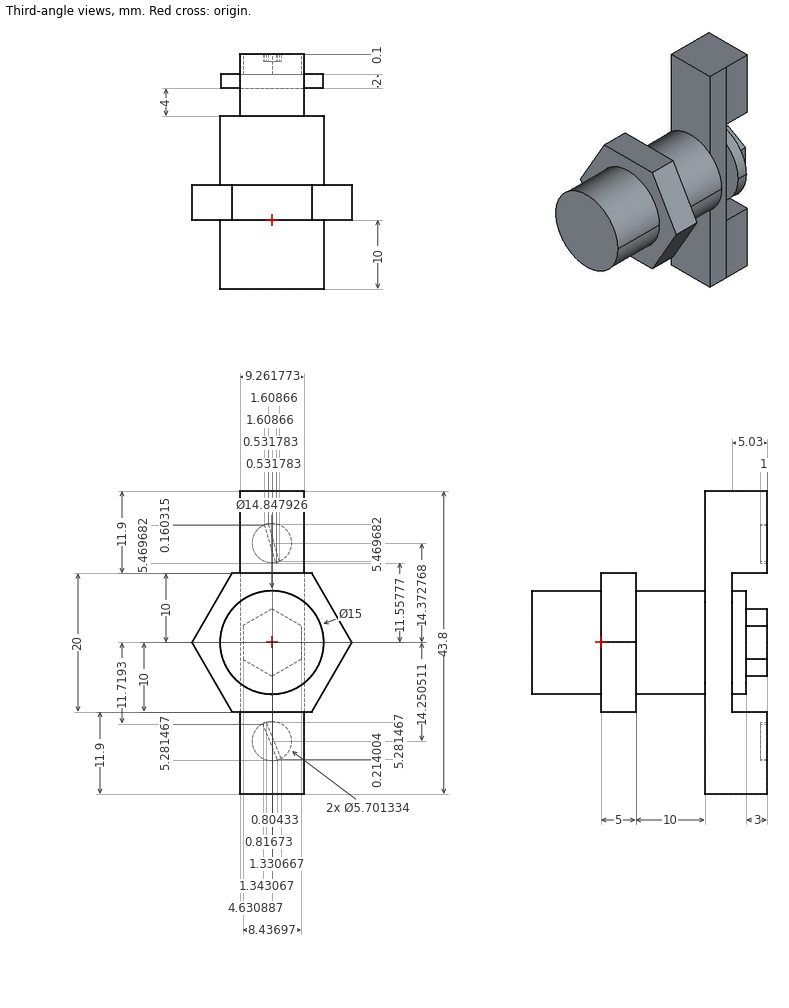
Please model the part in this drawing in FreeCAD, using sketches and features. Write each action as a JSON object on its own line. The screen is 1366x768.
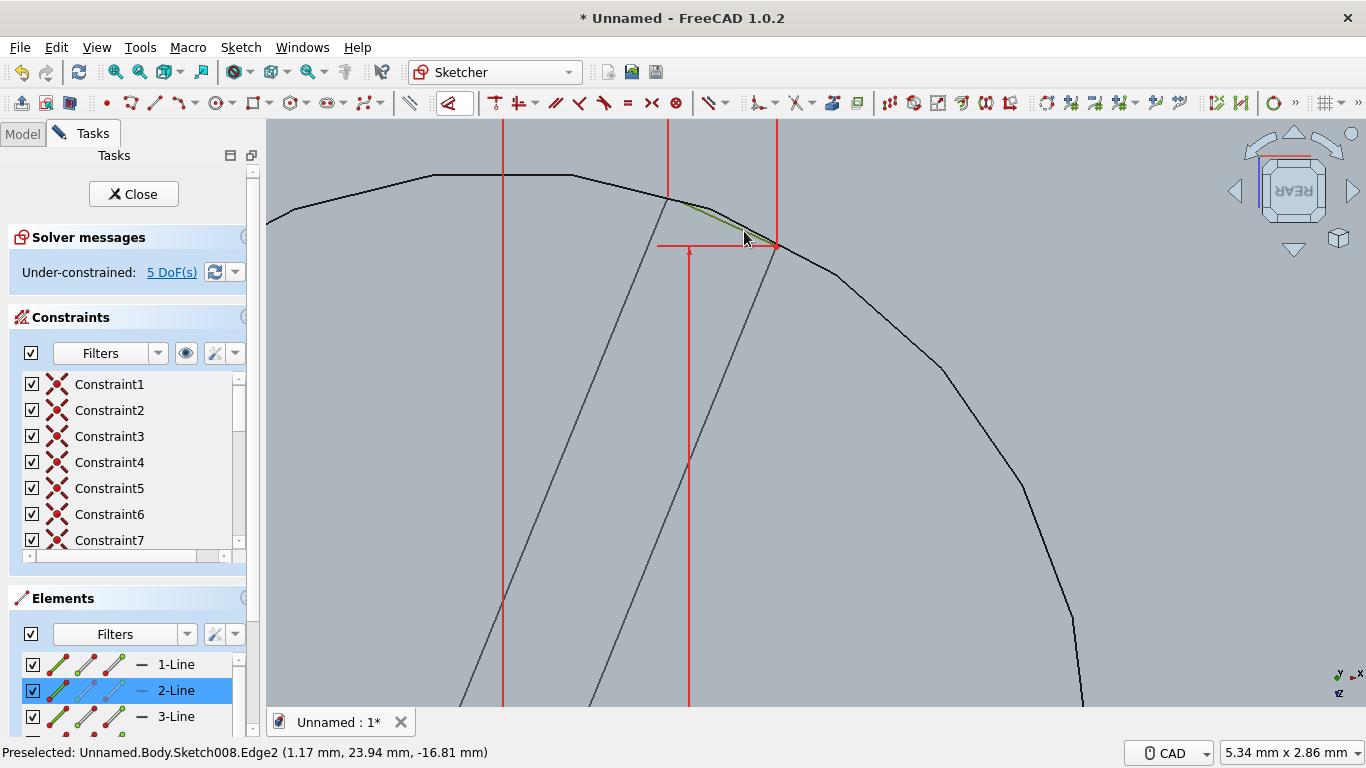
{"action": "left_click", "coordinate": [468, 104]}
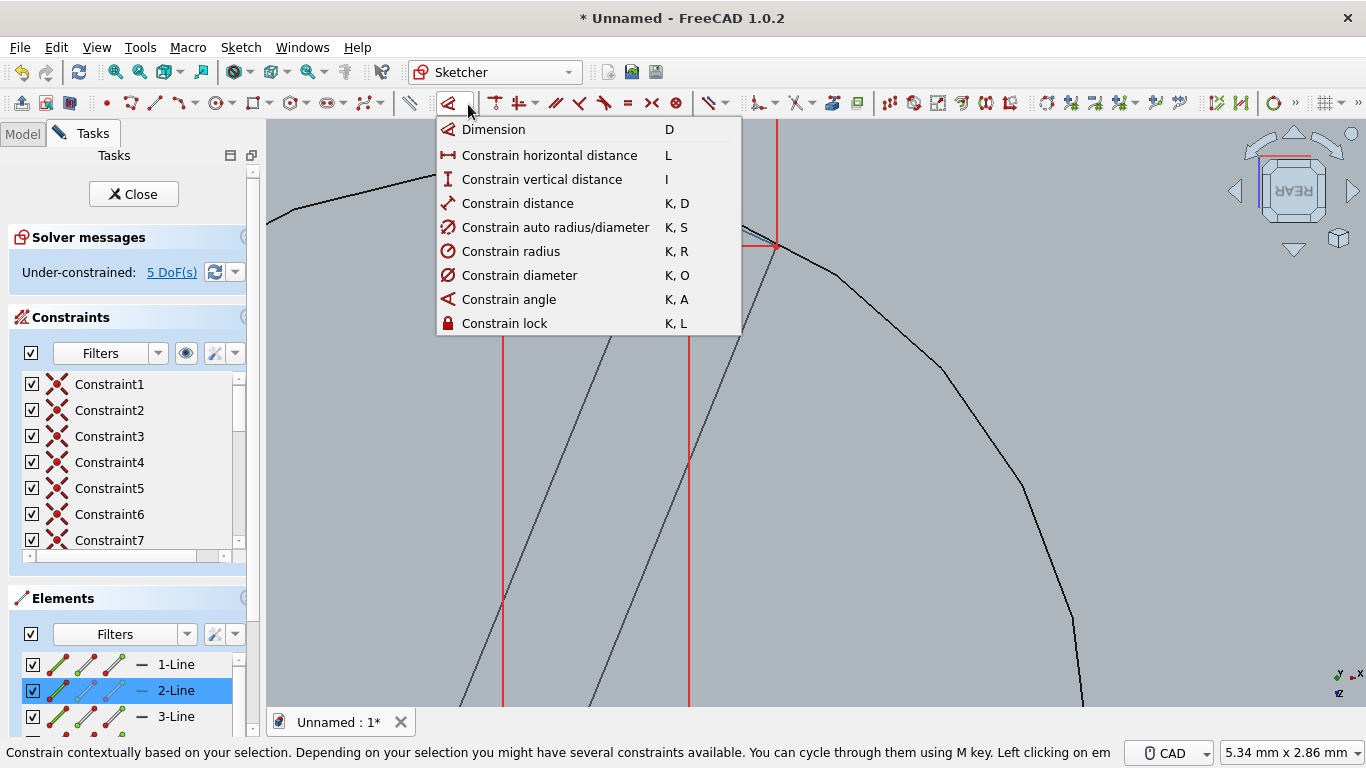
{"action": "left_click", "coordinate": [589, 179]}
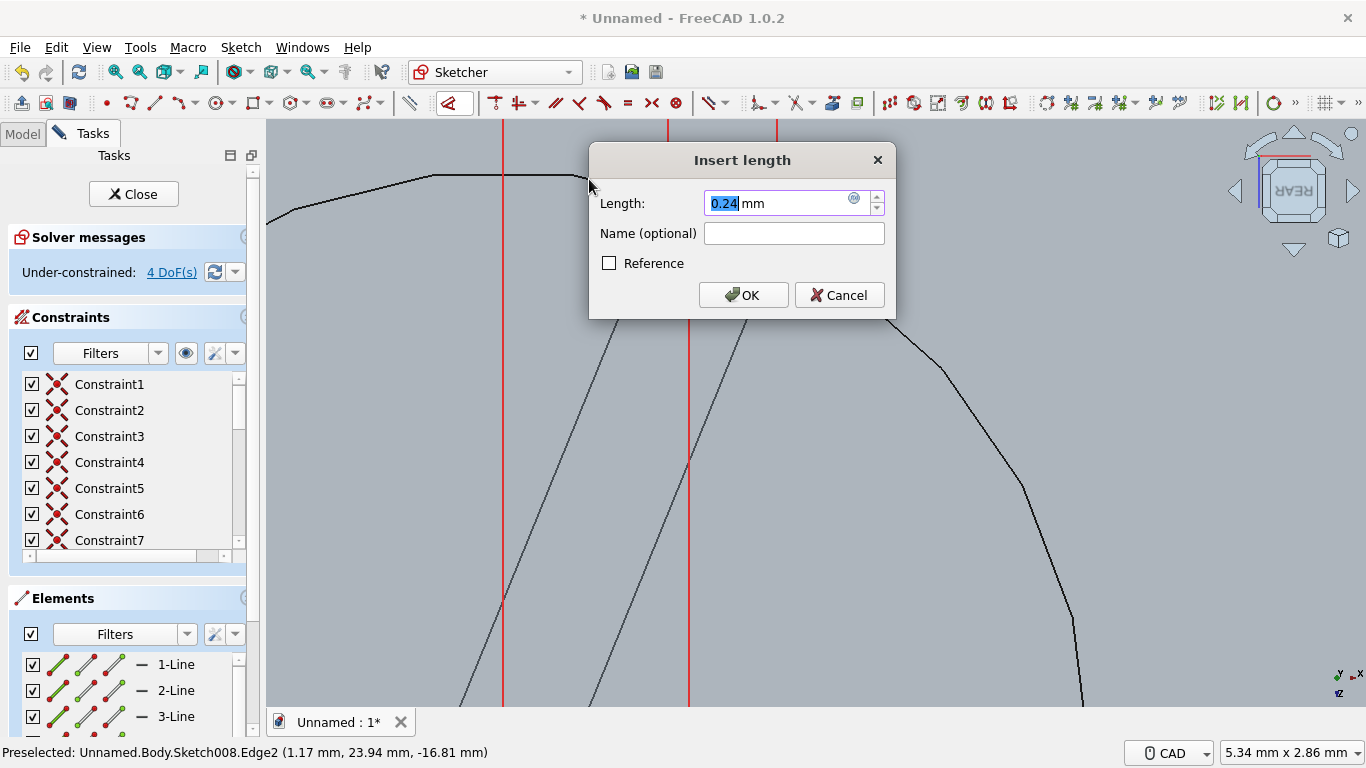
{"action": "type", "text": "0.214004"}
{"action": "key", "text": "Return"}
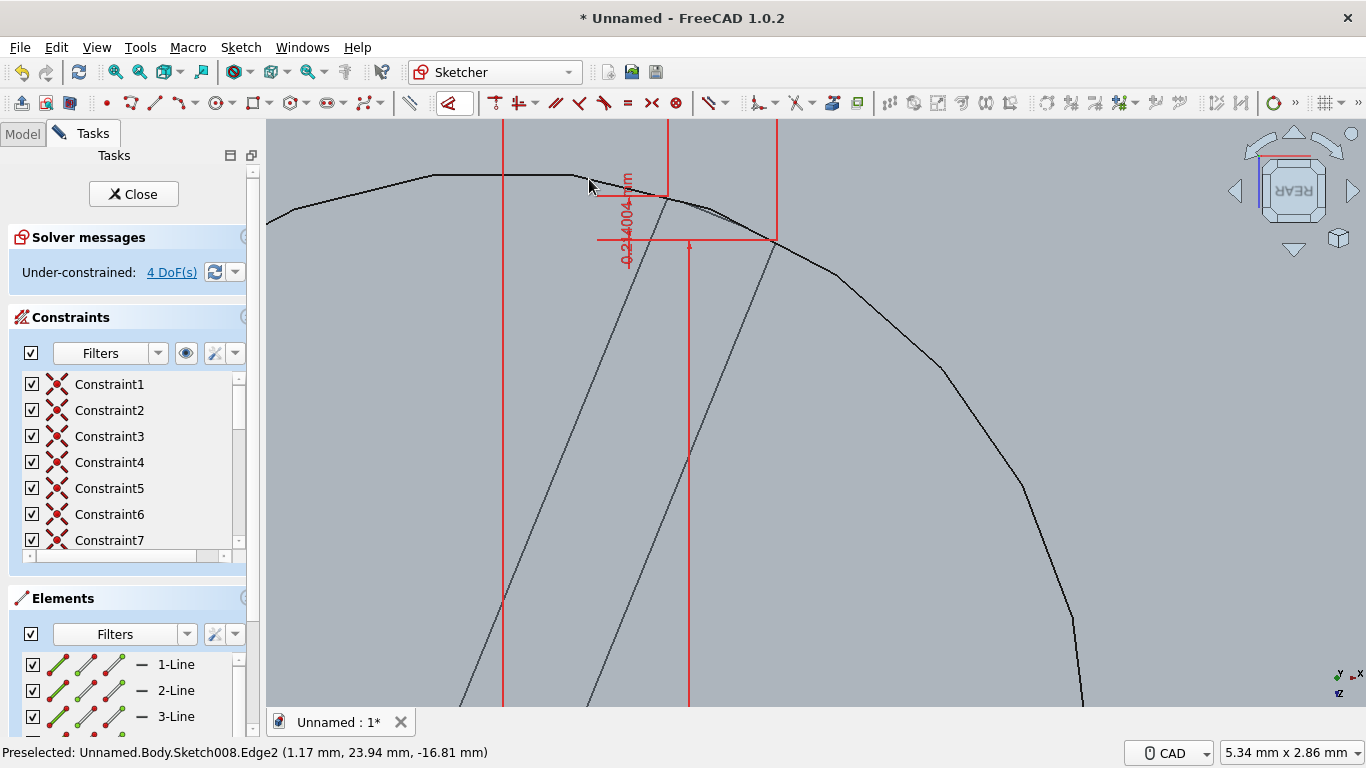
{"action": "left_click", "coordinate": [536, 521]}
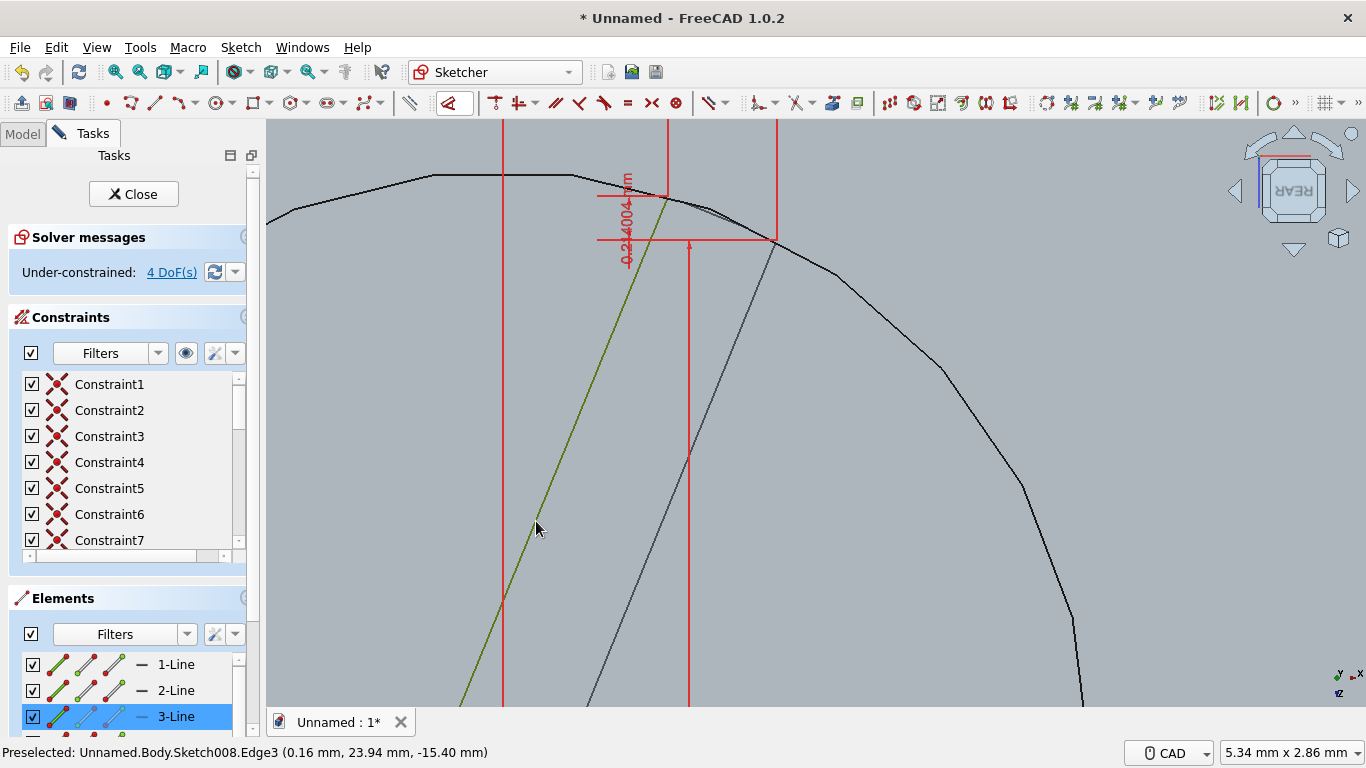
{"action": "key", "text": "i"}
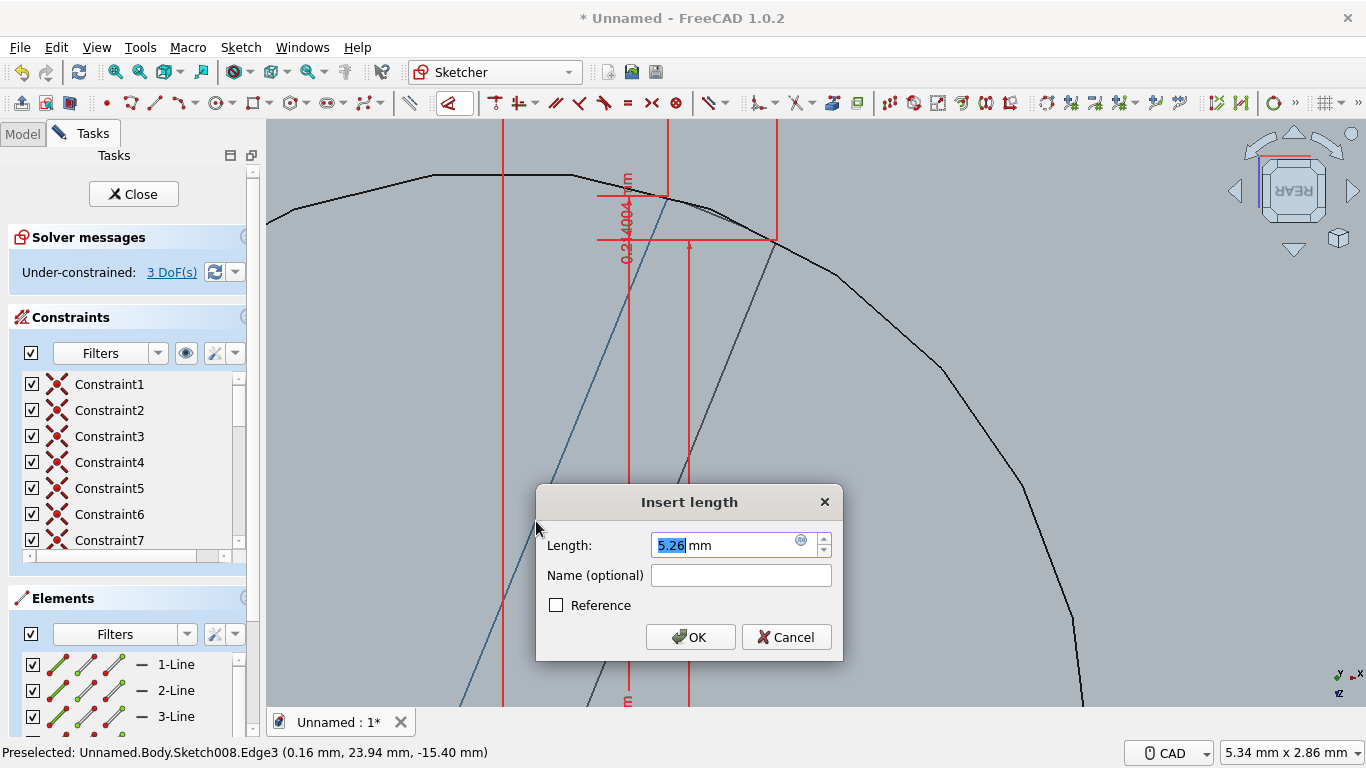
{"action": "type", "text": "5.281467"}
{"action": "key", "text": "Return"}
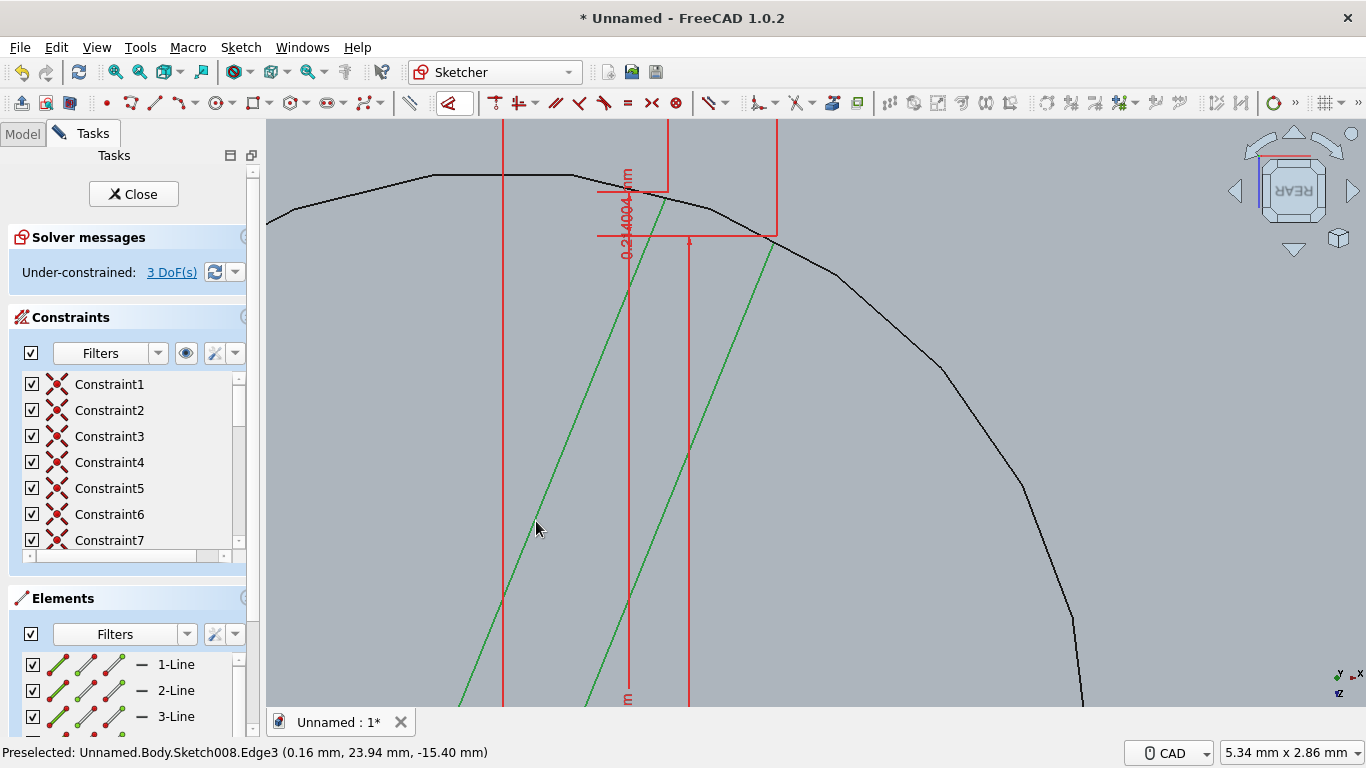
{"action": "scroll", "coordinate": [760, 240], "scroll_direction": "down", "scroll_amount": 15}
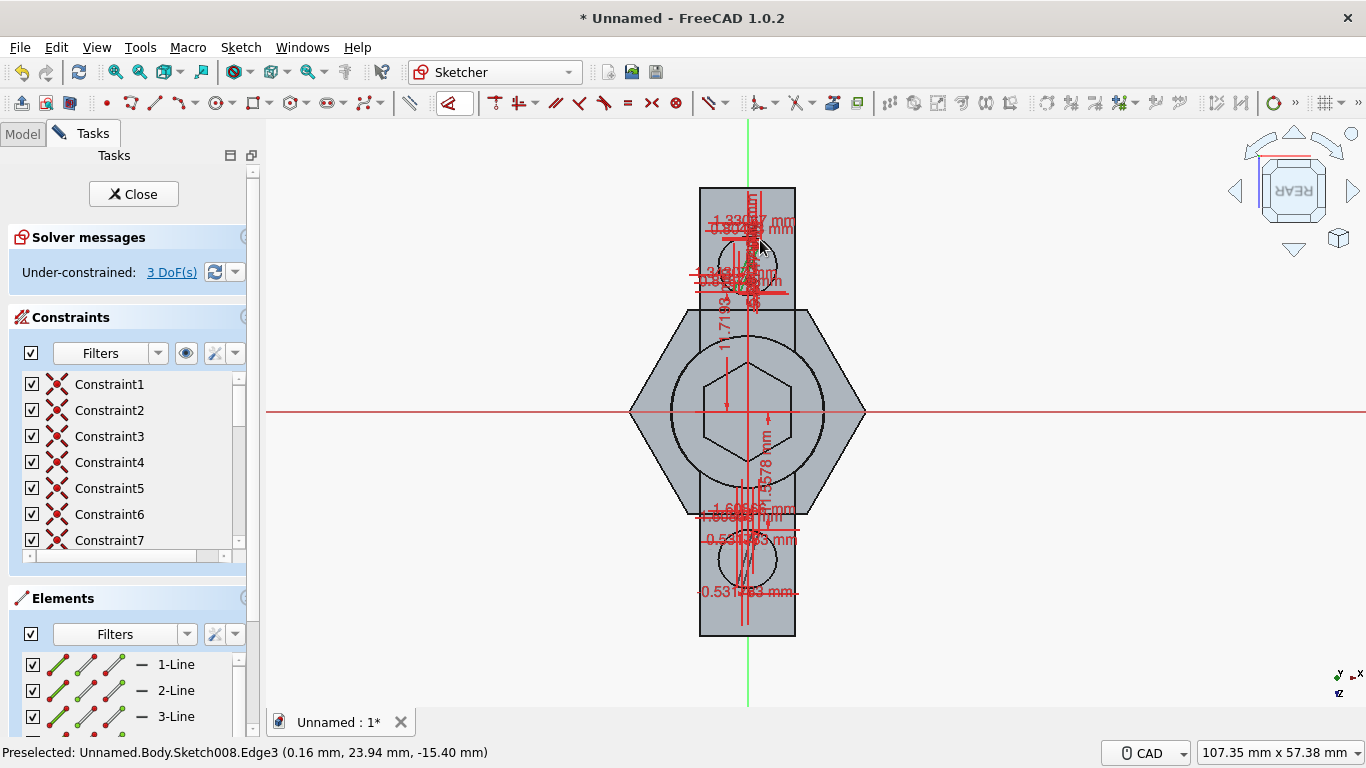
{"action": "scroll", "coordinate": [748, 547], "scroll_direction": "up", "scroll_amount": 14}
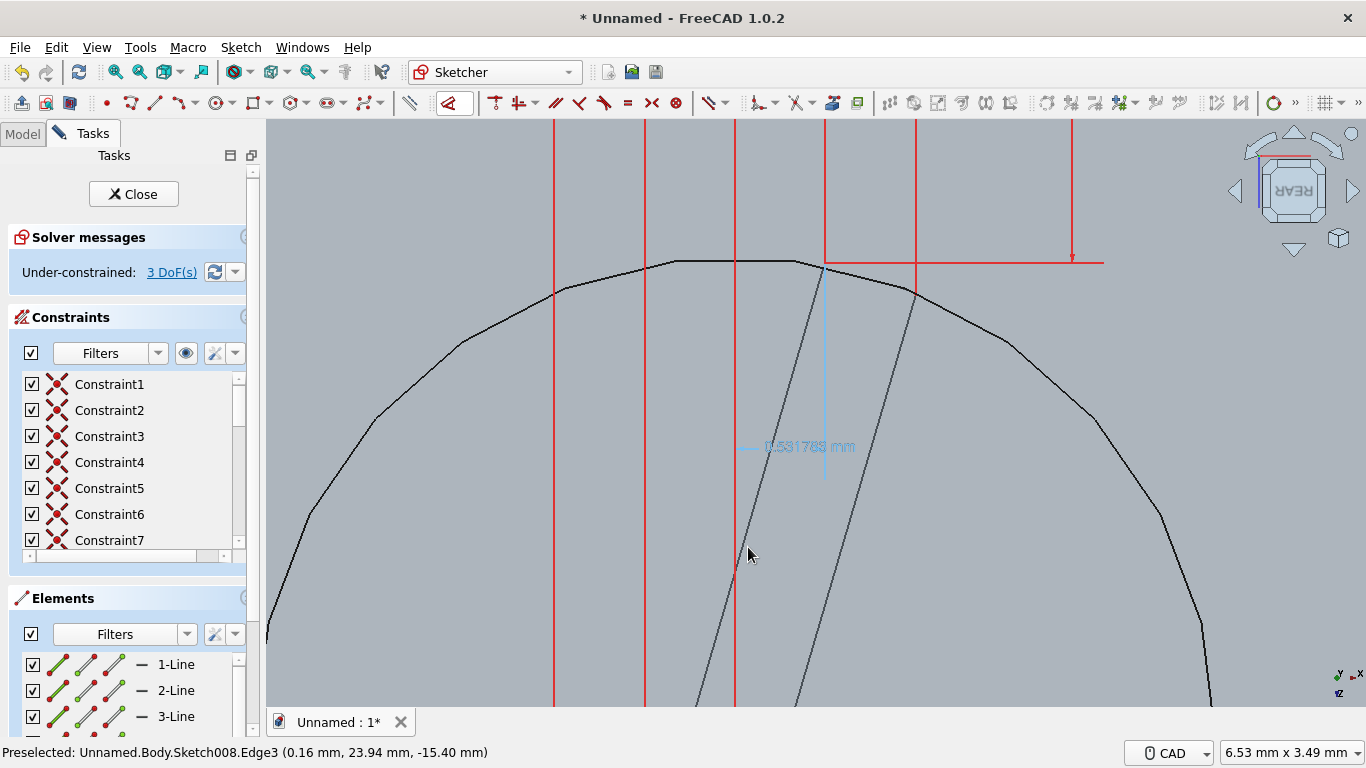
{"action": "left_click", "coordinate": [743, 544]}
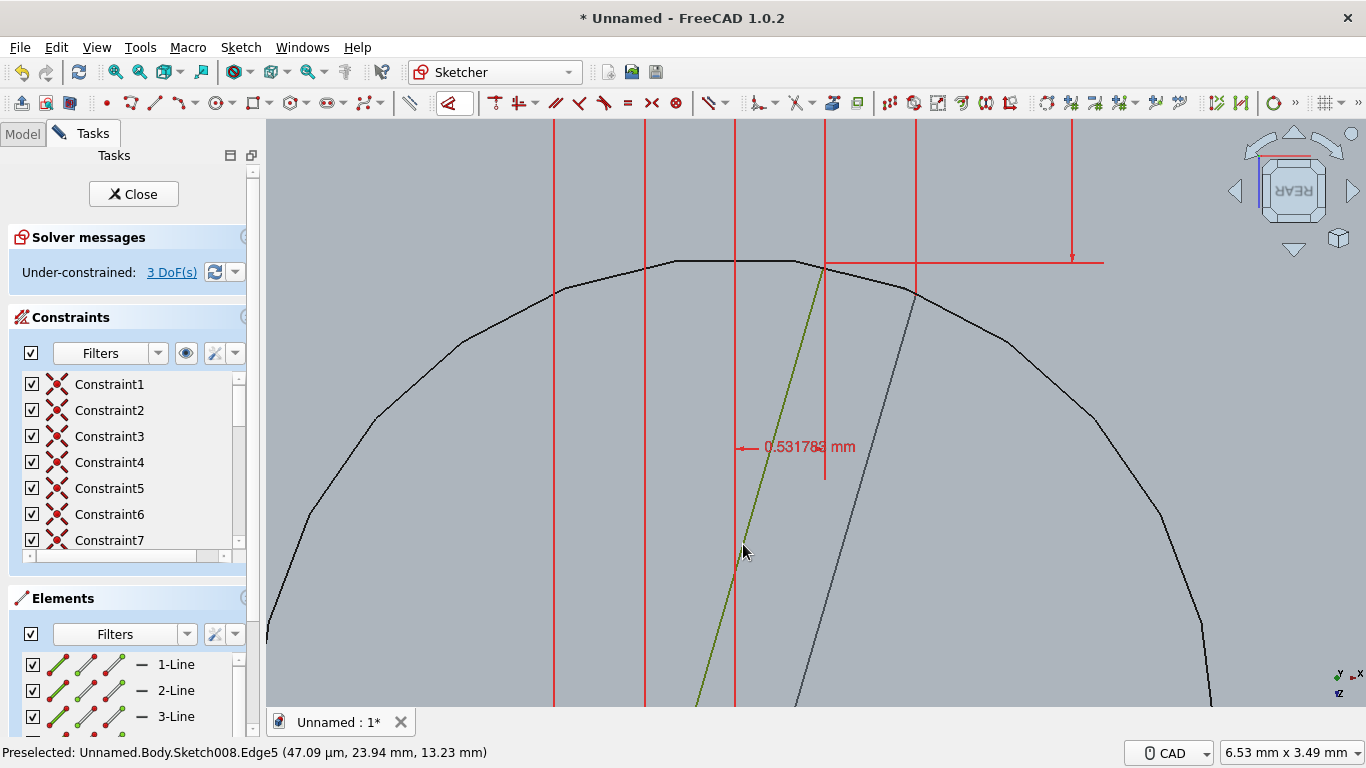
{"action": "key", "text": "i"}